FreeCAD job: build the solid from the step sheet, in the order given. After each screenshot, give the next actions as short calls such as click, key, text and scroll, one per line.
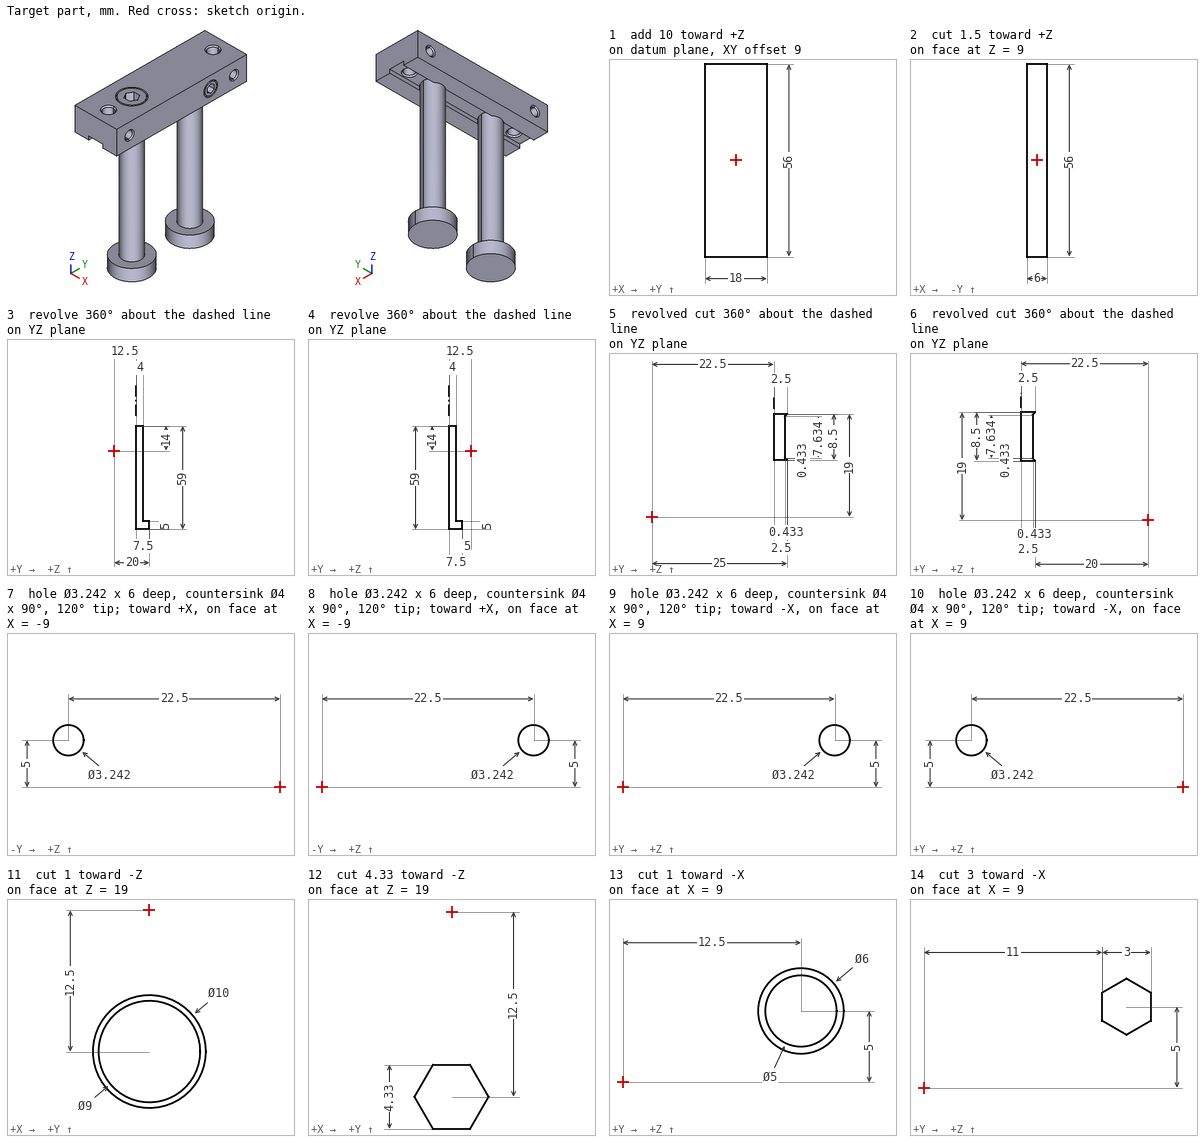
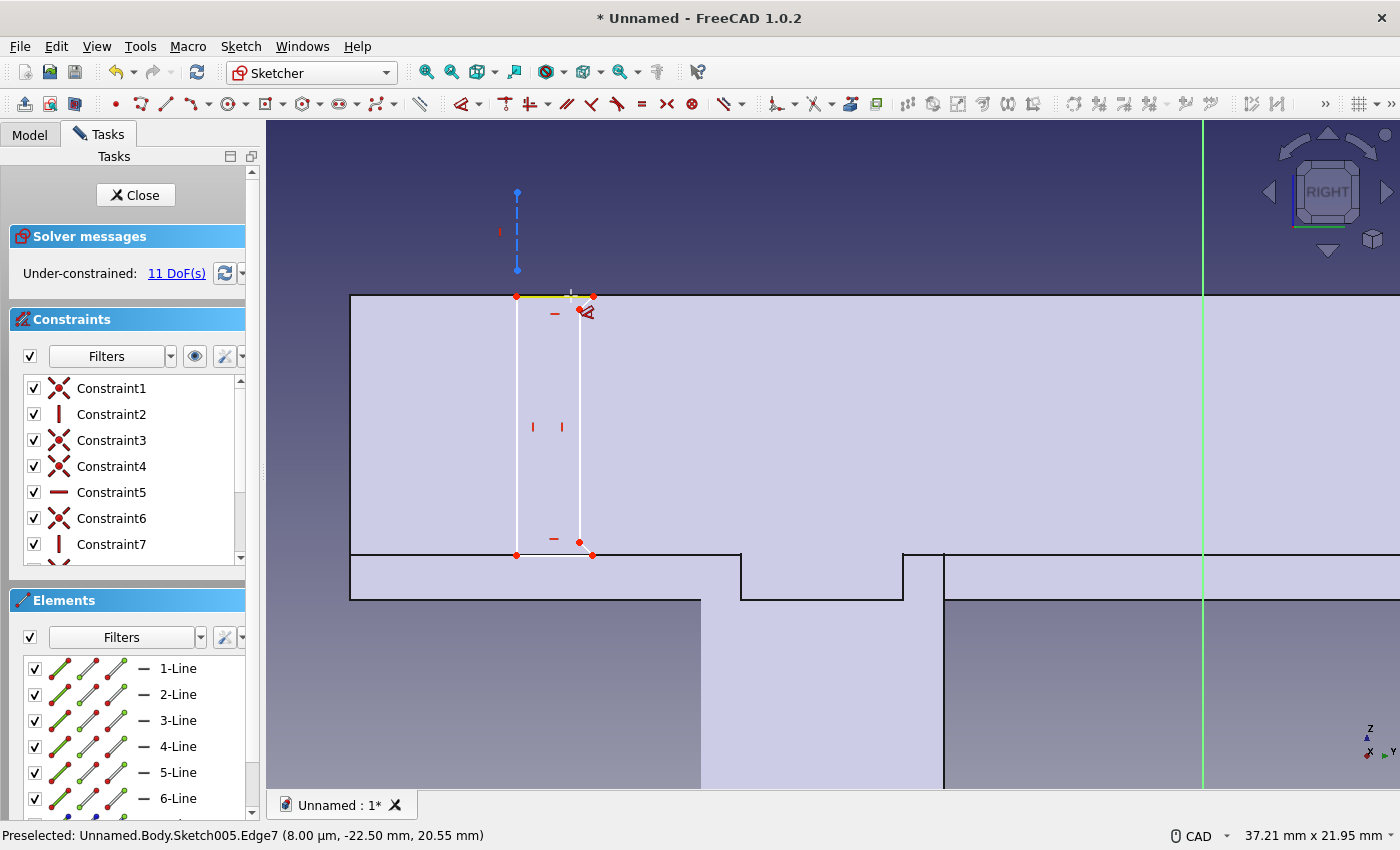
click(571, 297)
click(555, 263)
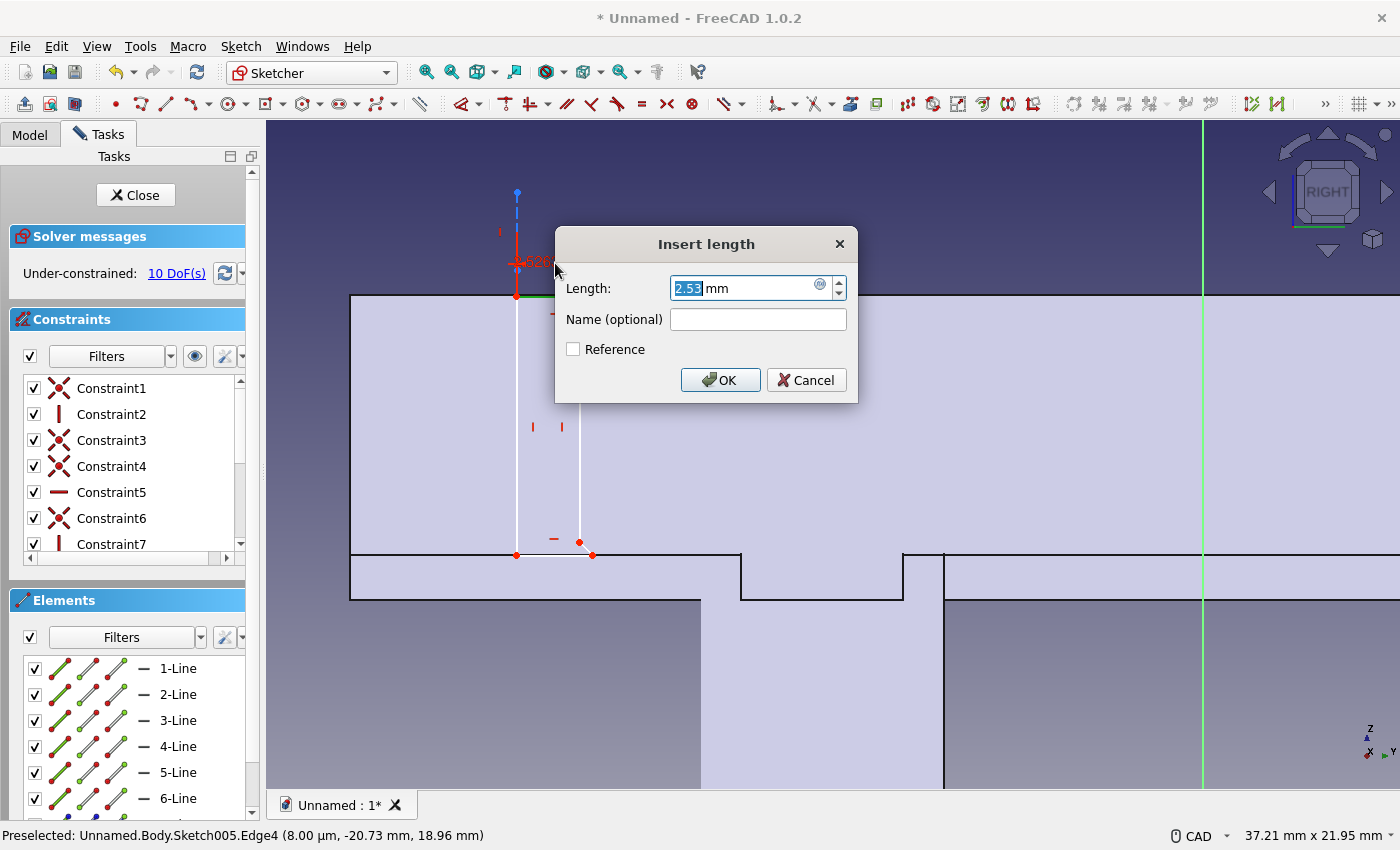
text(2.5)
key(Return)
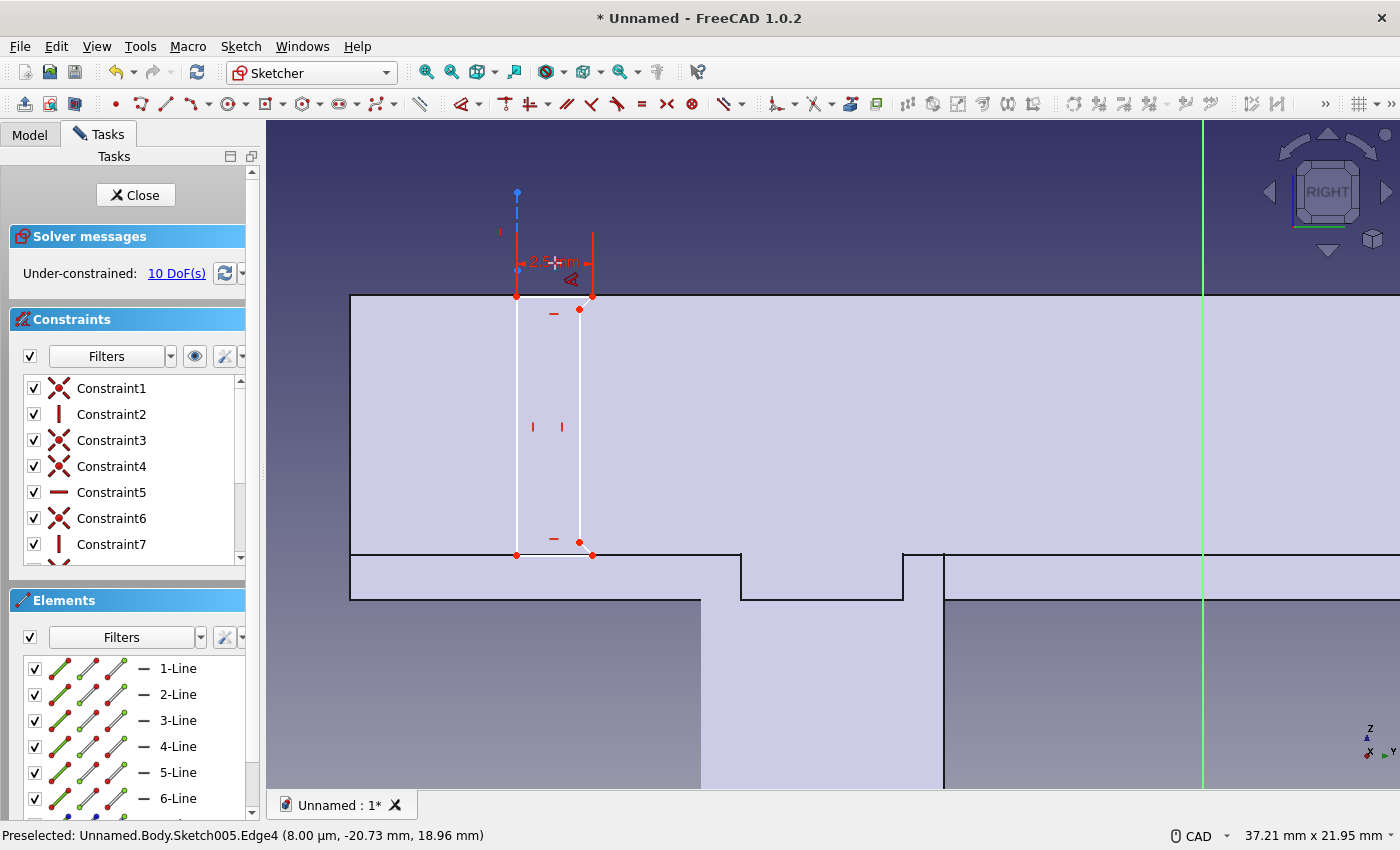
click(517, 374)
click(483, 426)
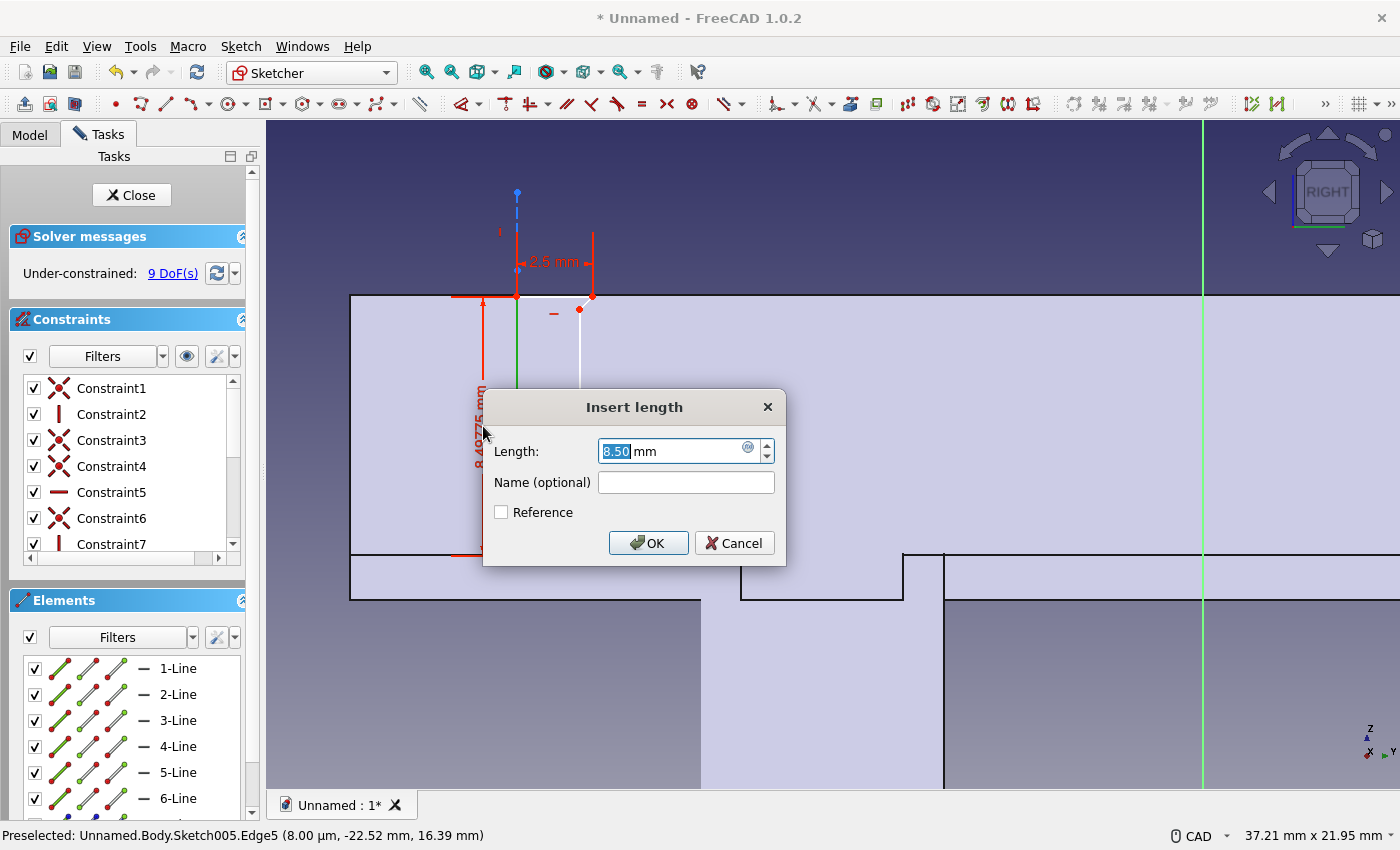
text(8.5)
key(Return)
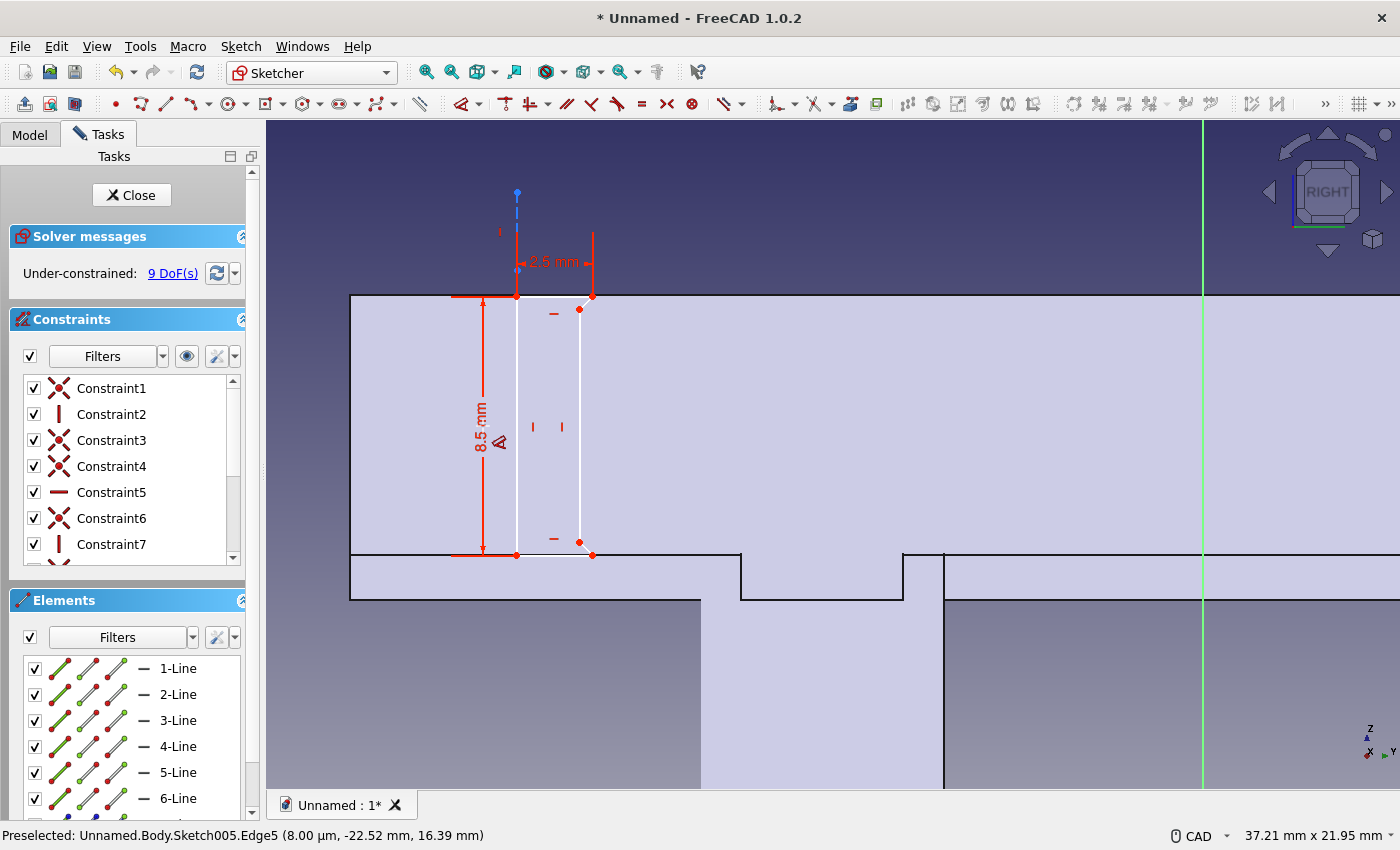
click(540, 556)
click(555, 590)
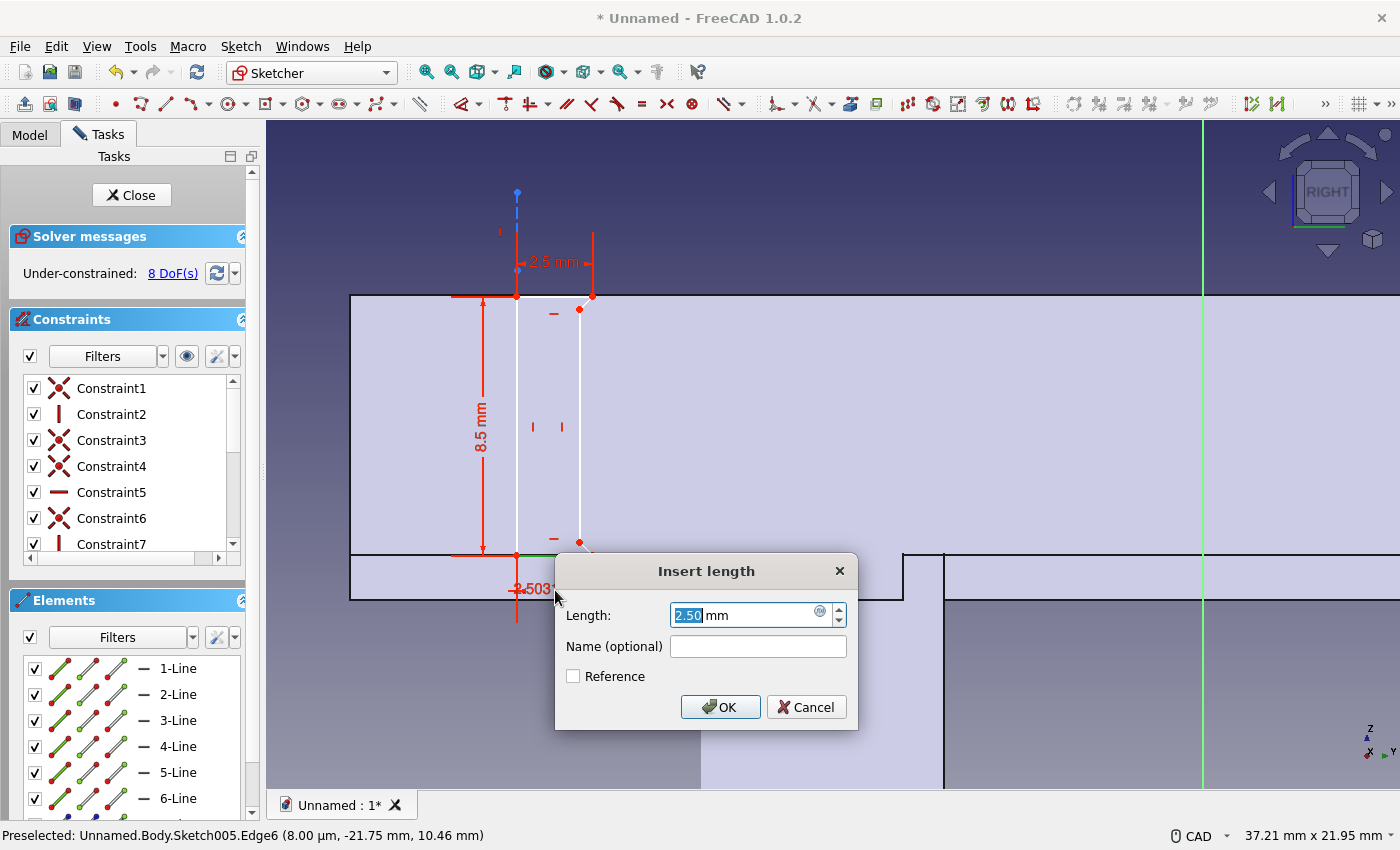
text(2.5)
key(Return)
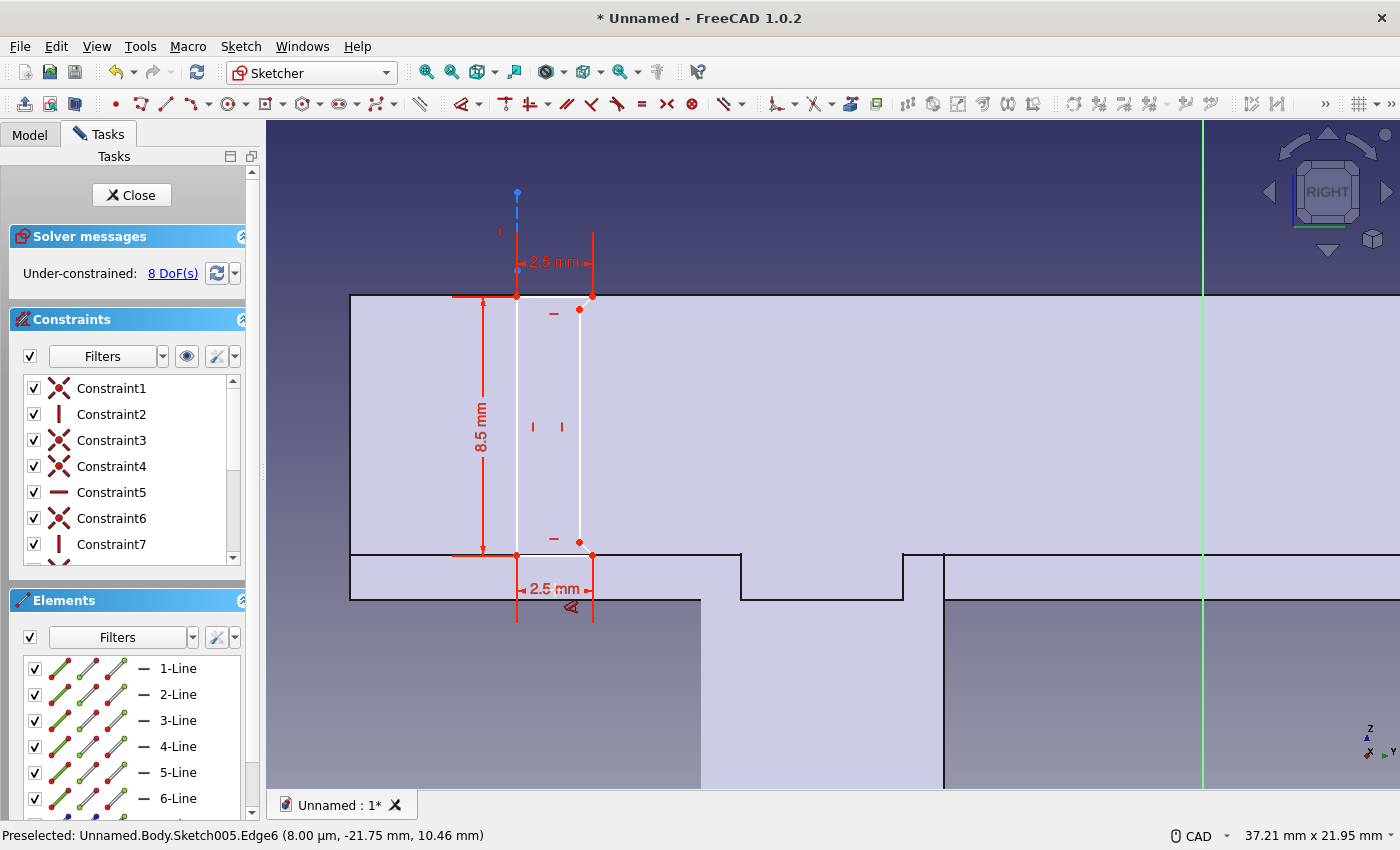
click(593, 556)
click(898, 522)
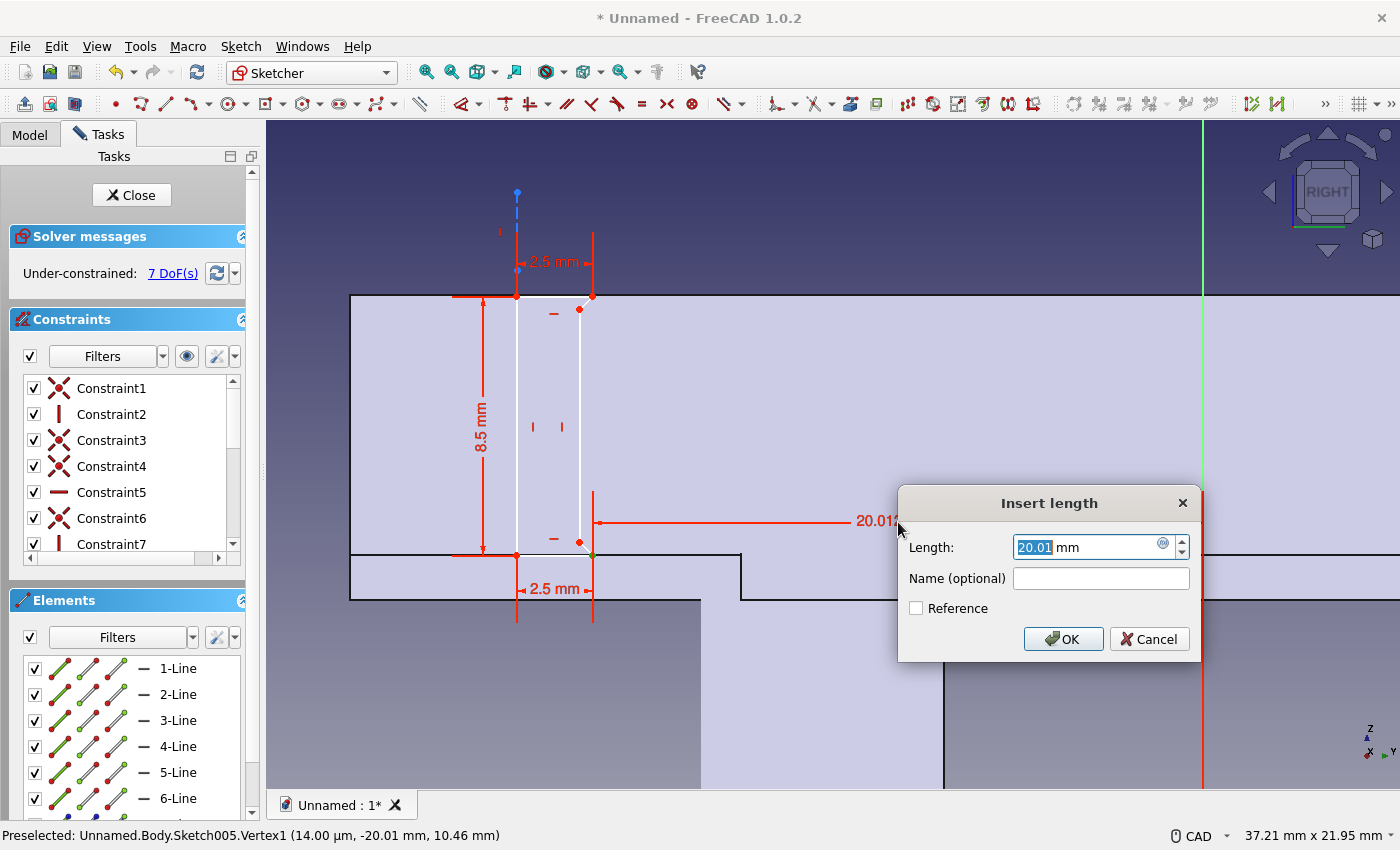
text(20)
key(Return)